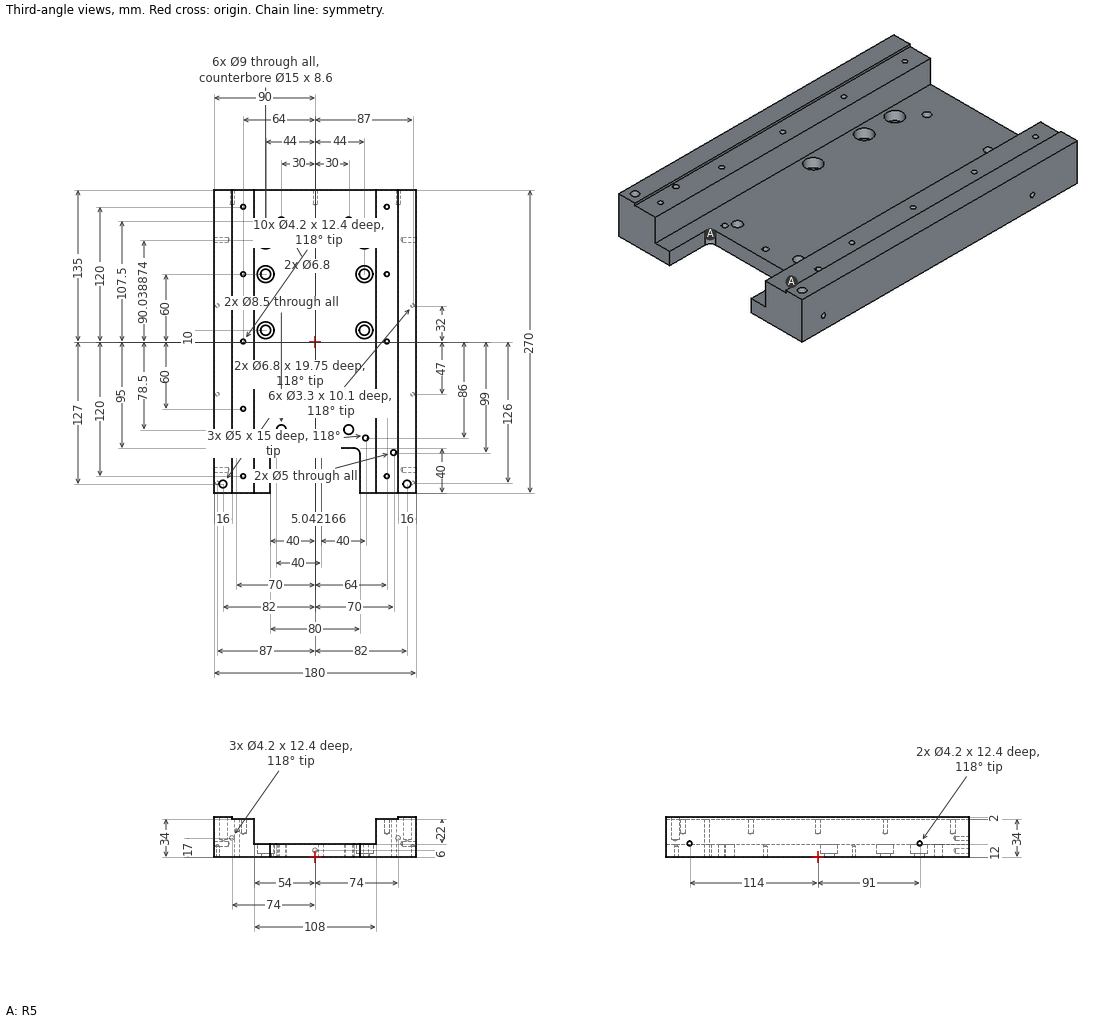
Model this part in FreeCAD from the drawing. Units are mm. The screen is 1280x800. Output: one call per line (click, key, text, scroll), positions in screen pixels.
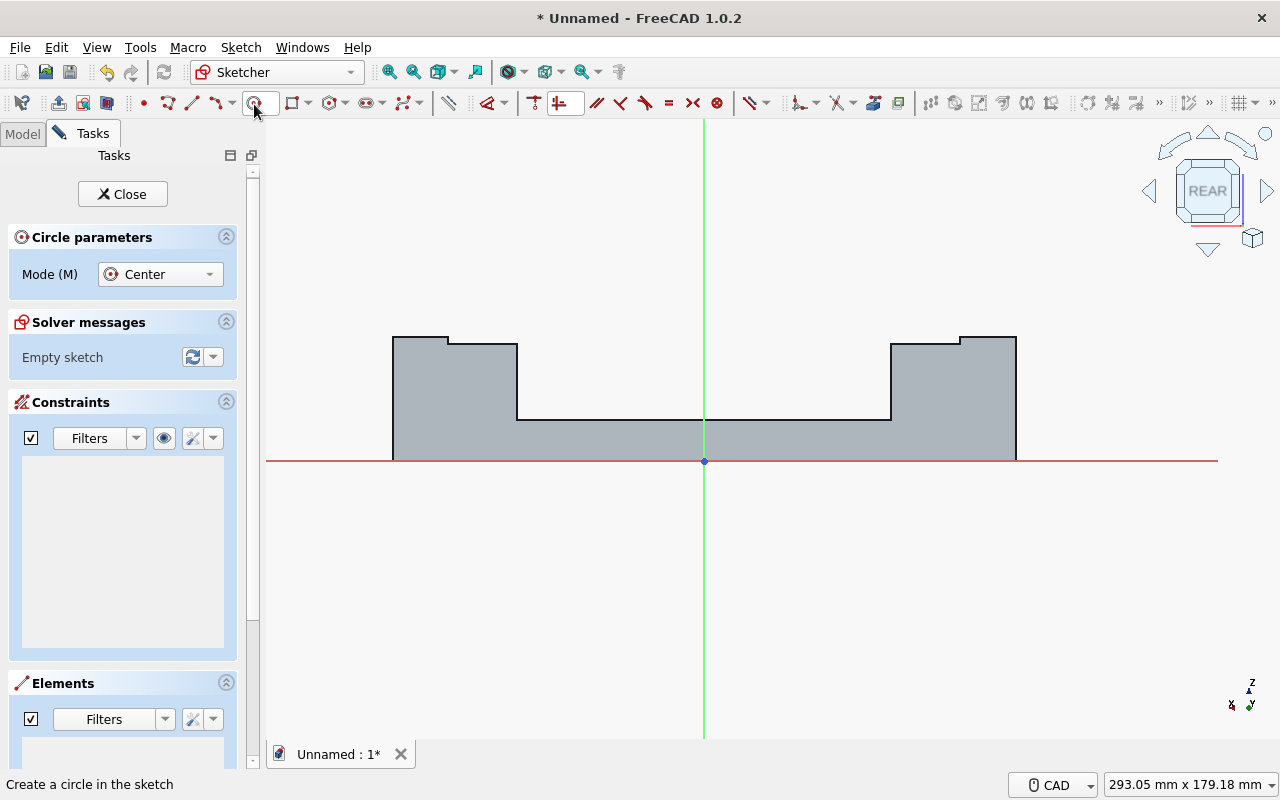
scroll(960, 402, up, 6)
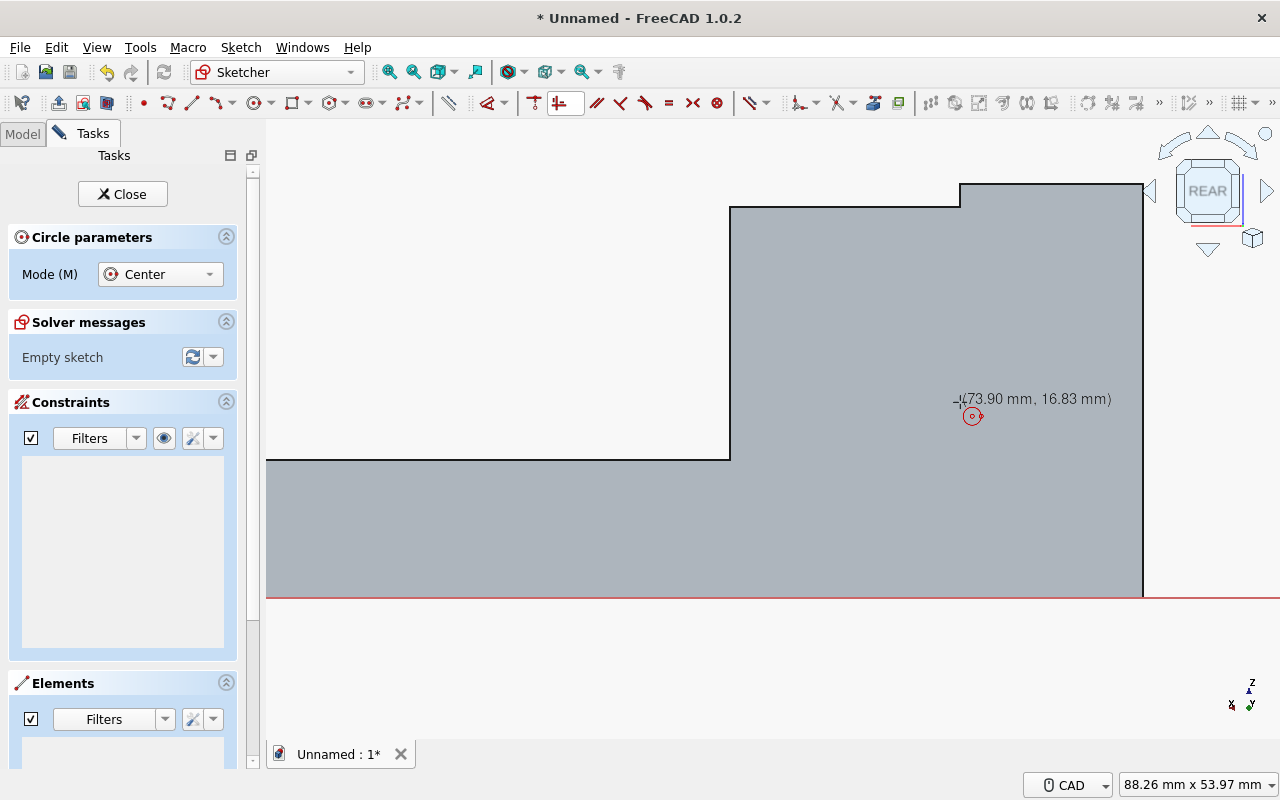
click(960, 402)
move(977, 385)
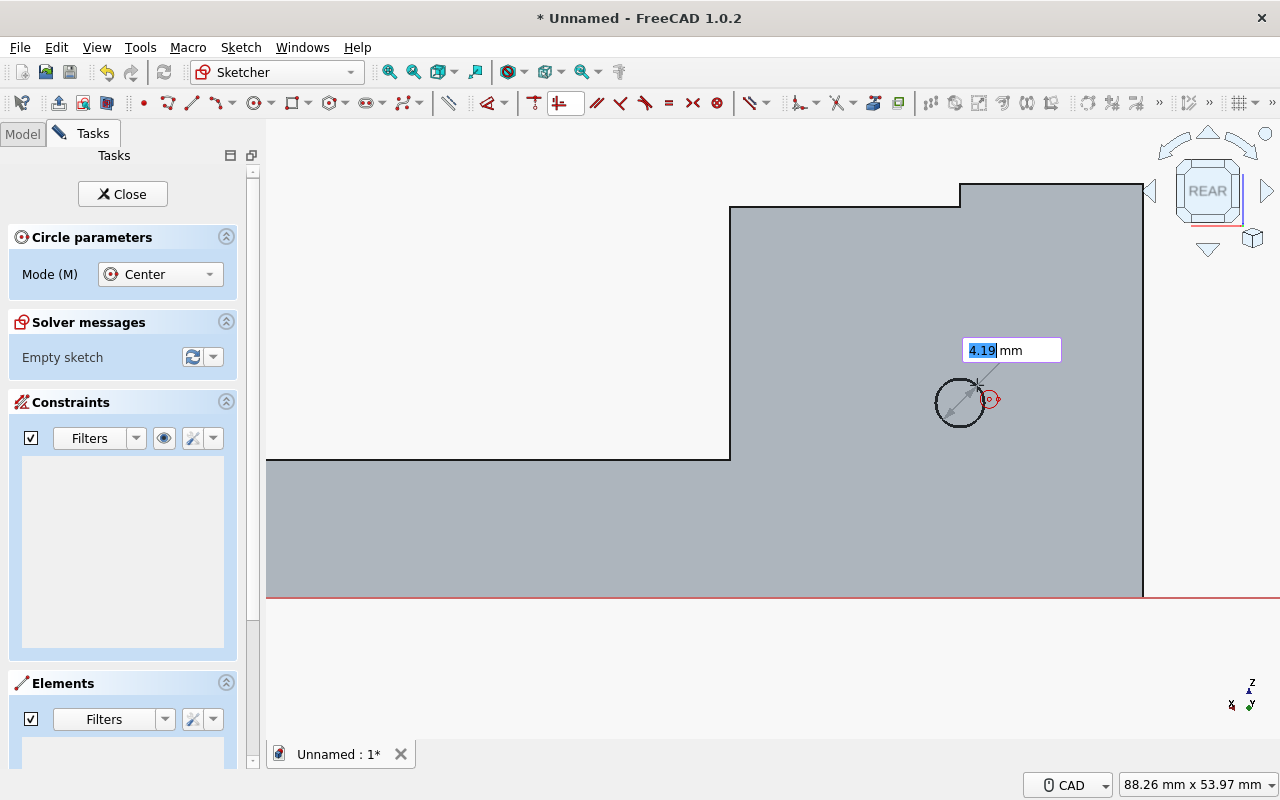
text(4.2)
key(Return)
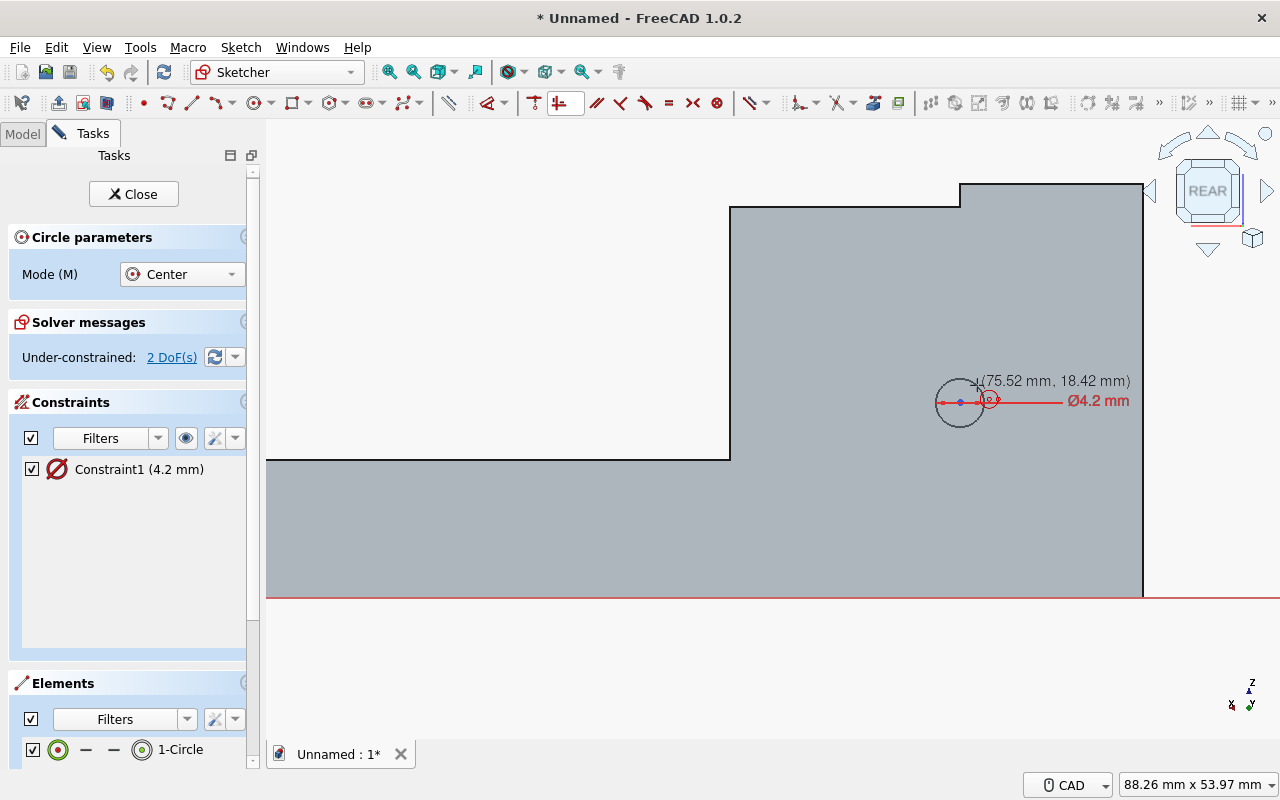
scroll(961, 404, down, 6)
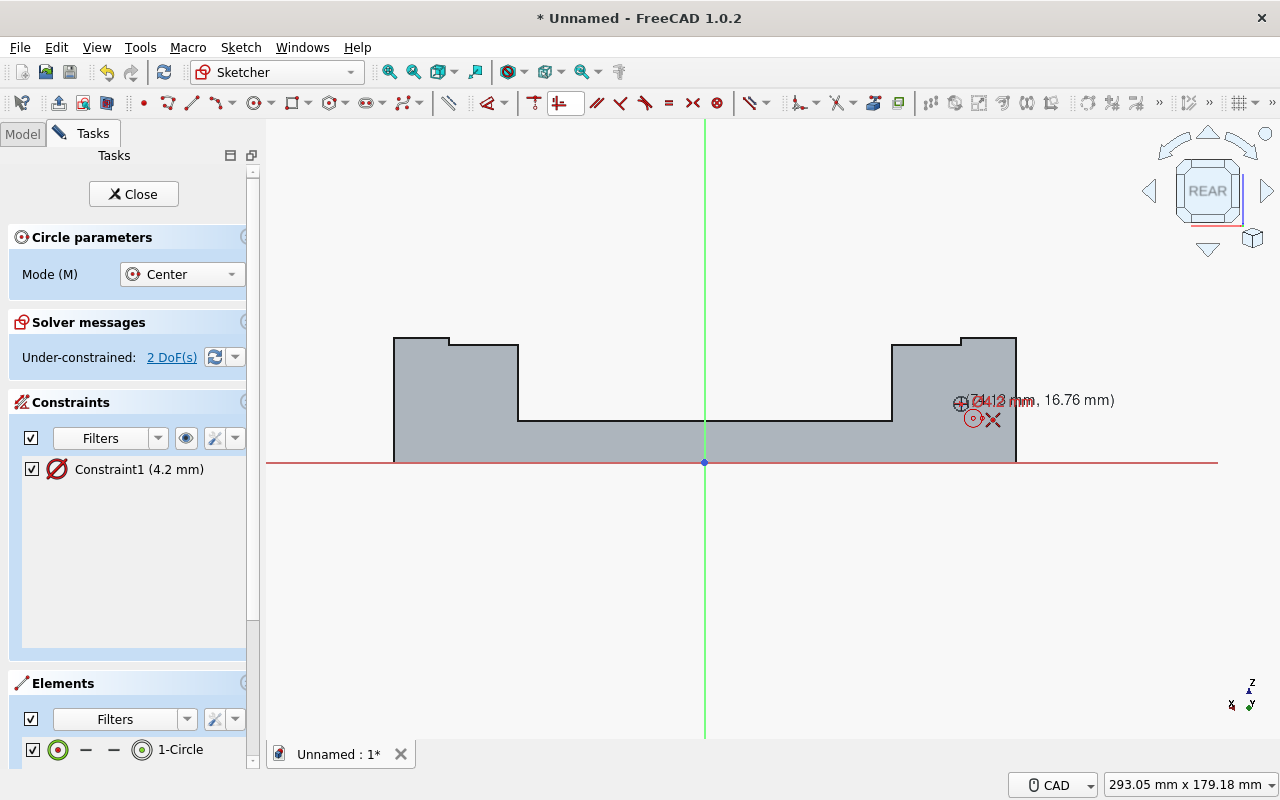
scroll(449, 404, up, 6)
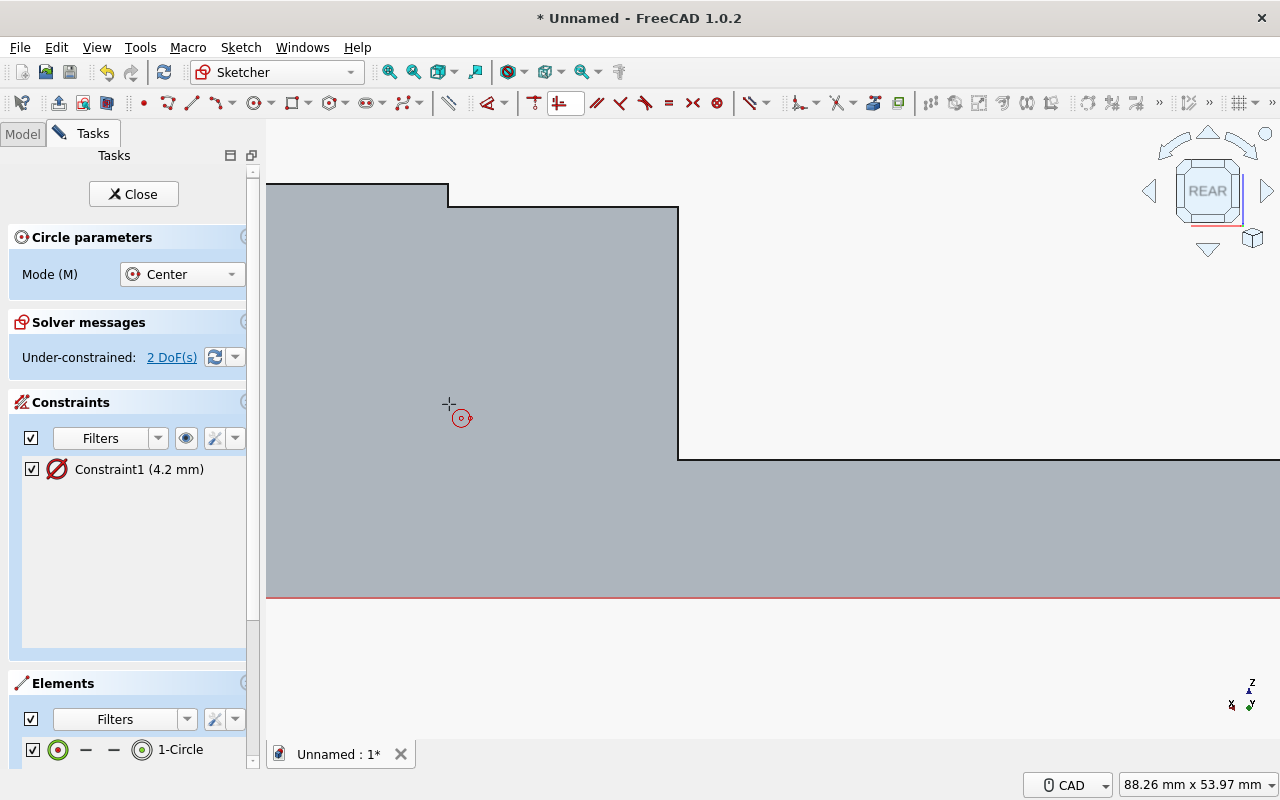
click(448, 402)
move(465, 385)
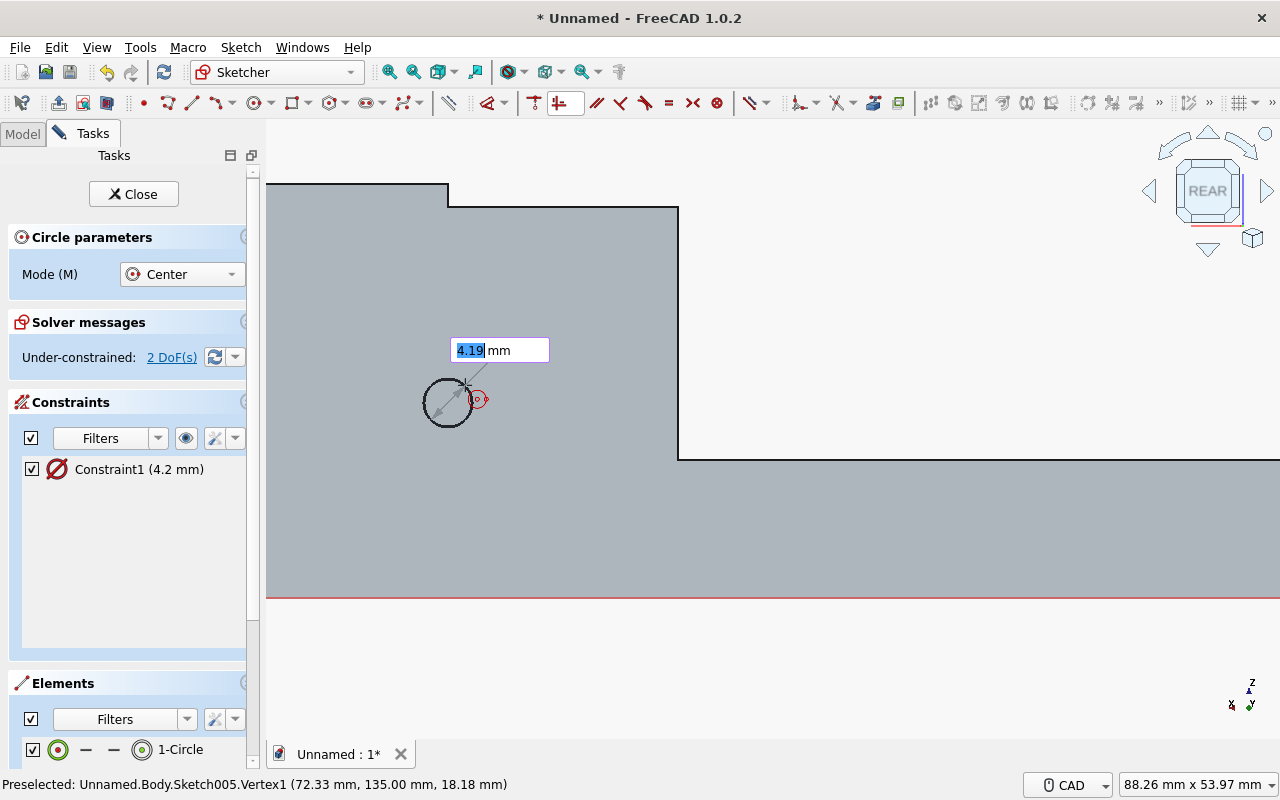
text(4.2)
key(Return)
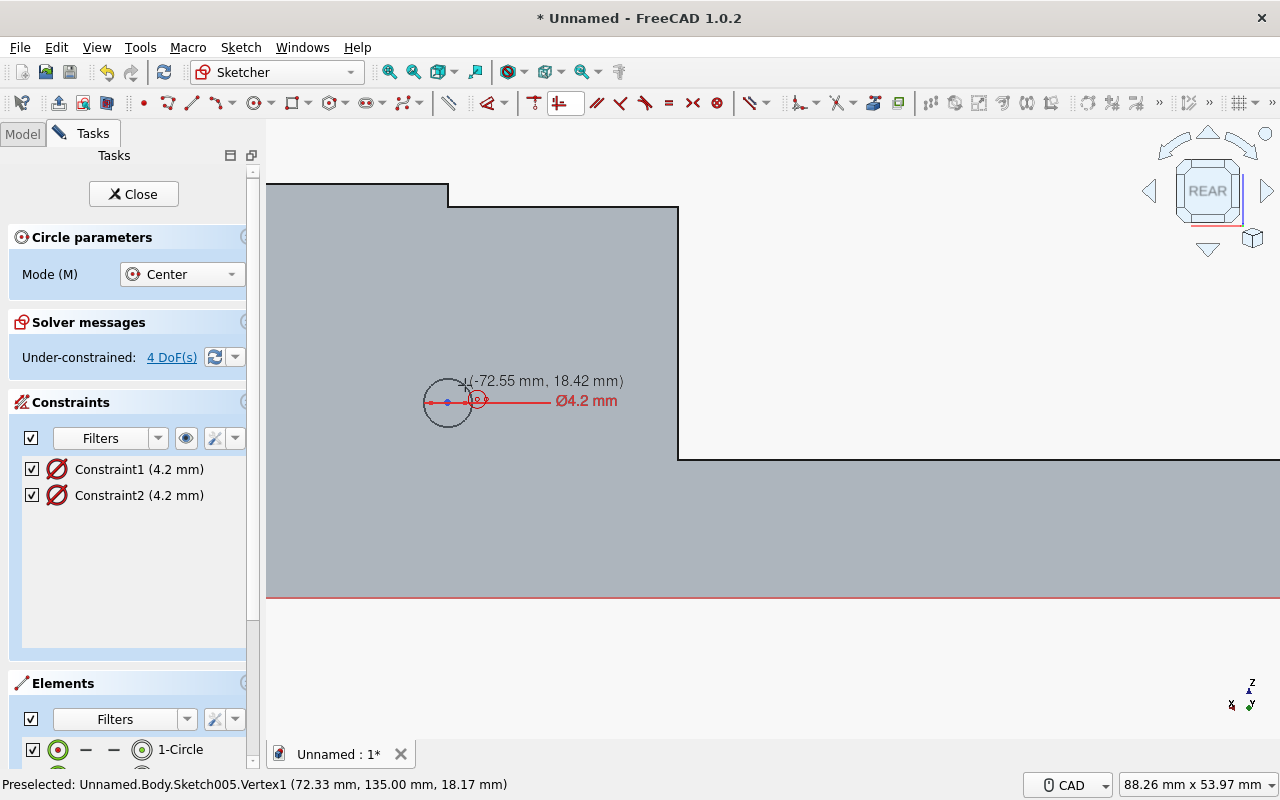
scroll(448, 404, down, 6)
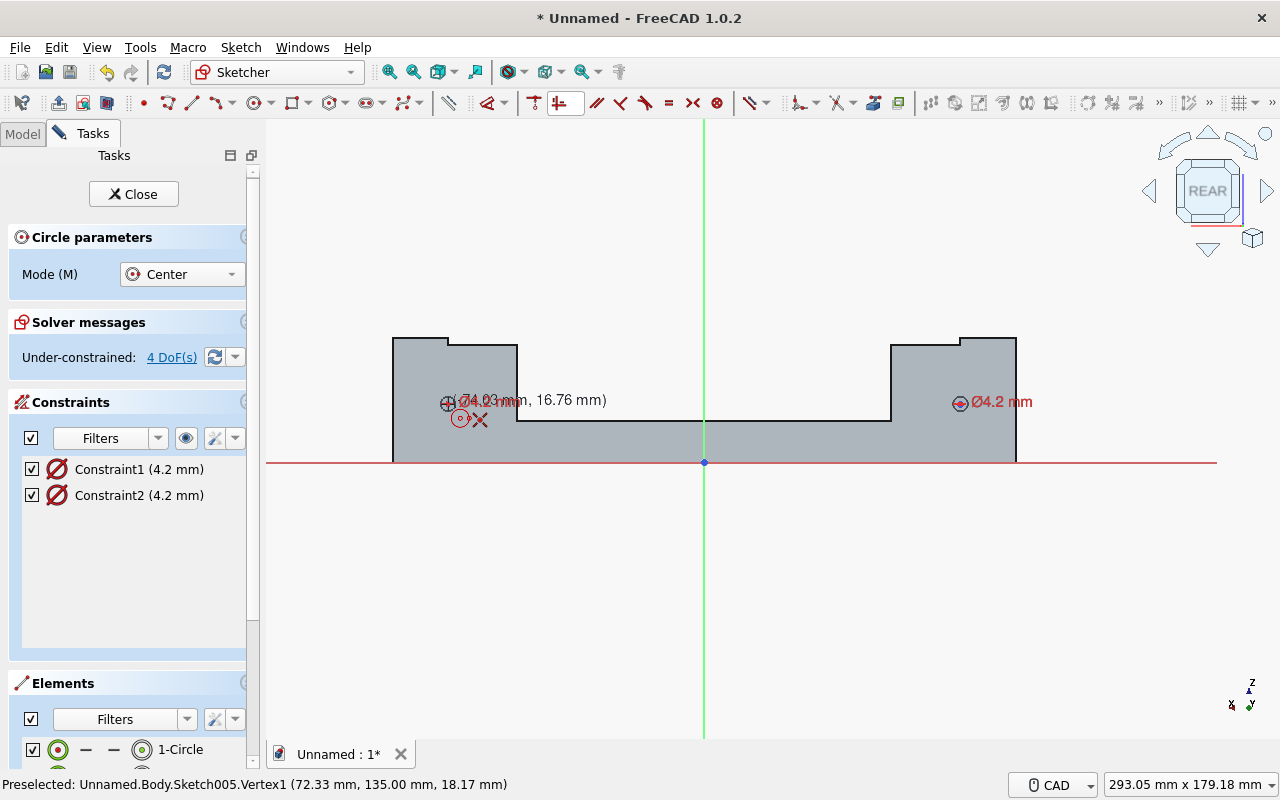
scroll(704, 442, up, 6)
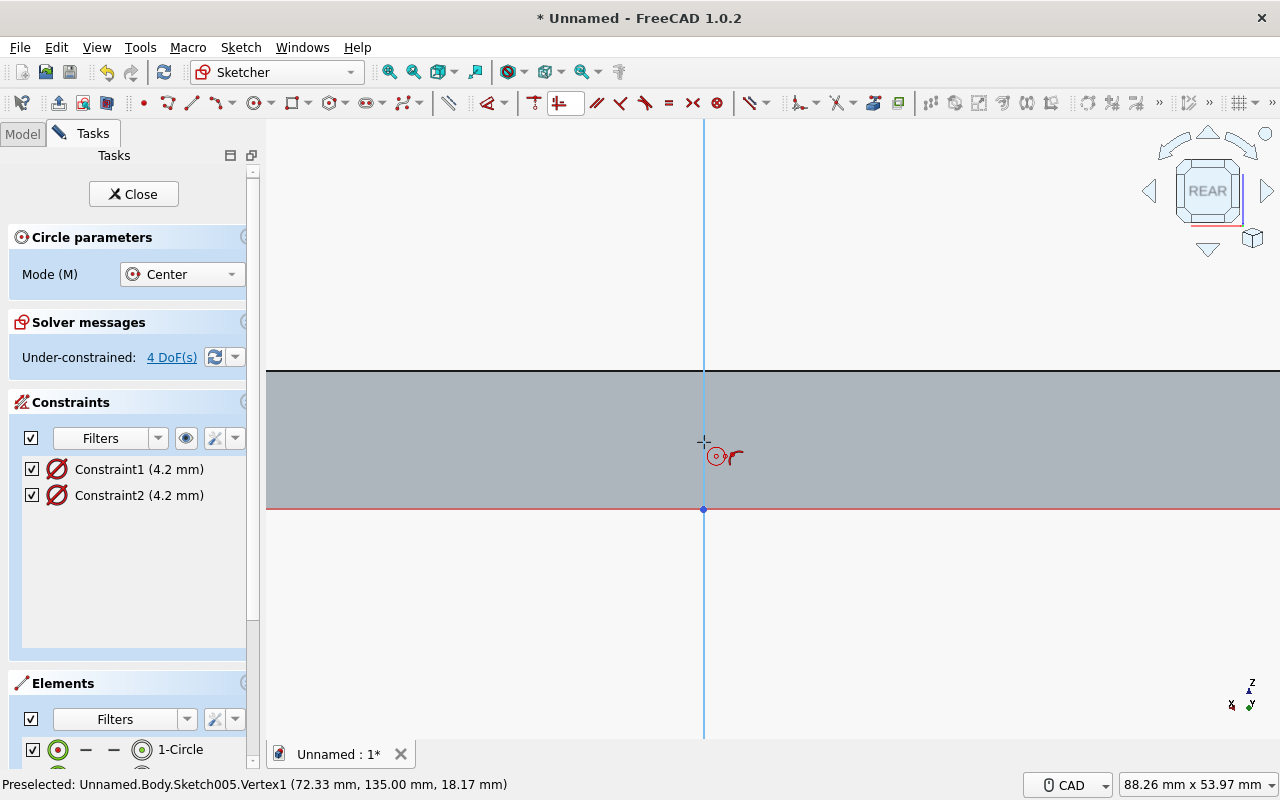
click(704, 440)
move(721, 423)